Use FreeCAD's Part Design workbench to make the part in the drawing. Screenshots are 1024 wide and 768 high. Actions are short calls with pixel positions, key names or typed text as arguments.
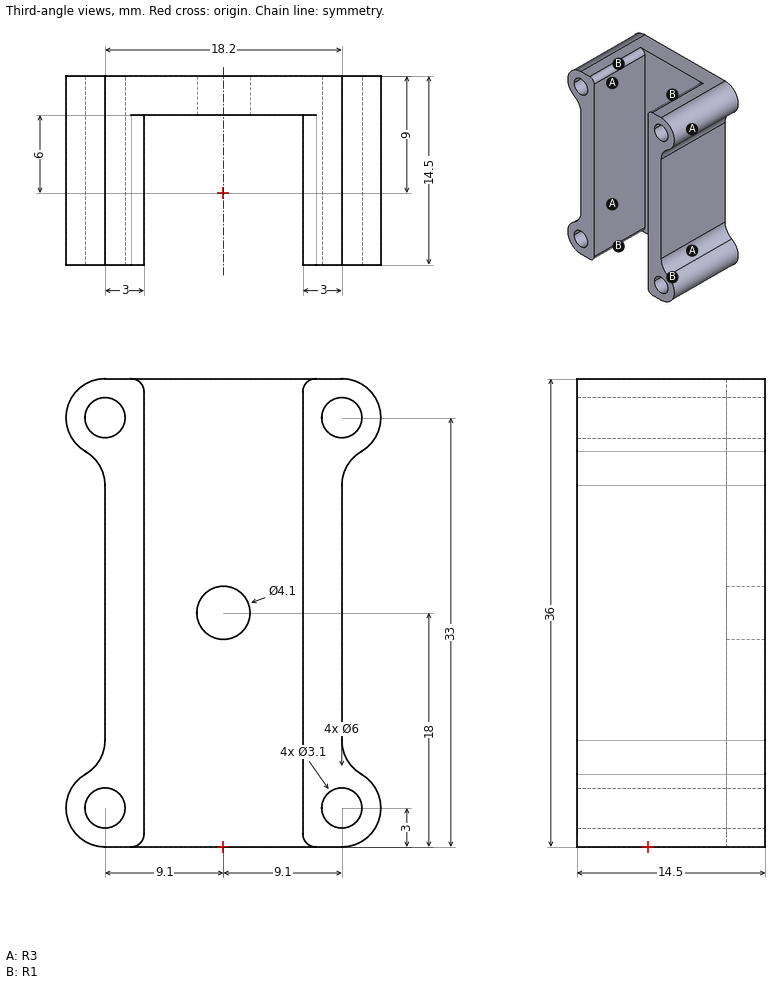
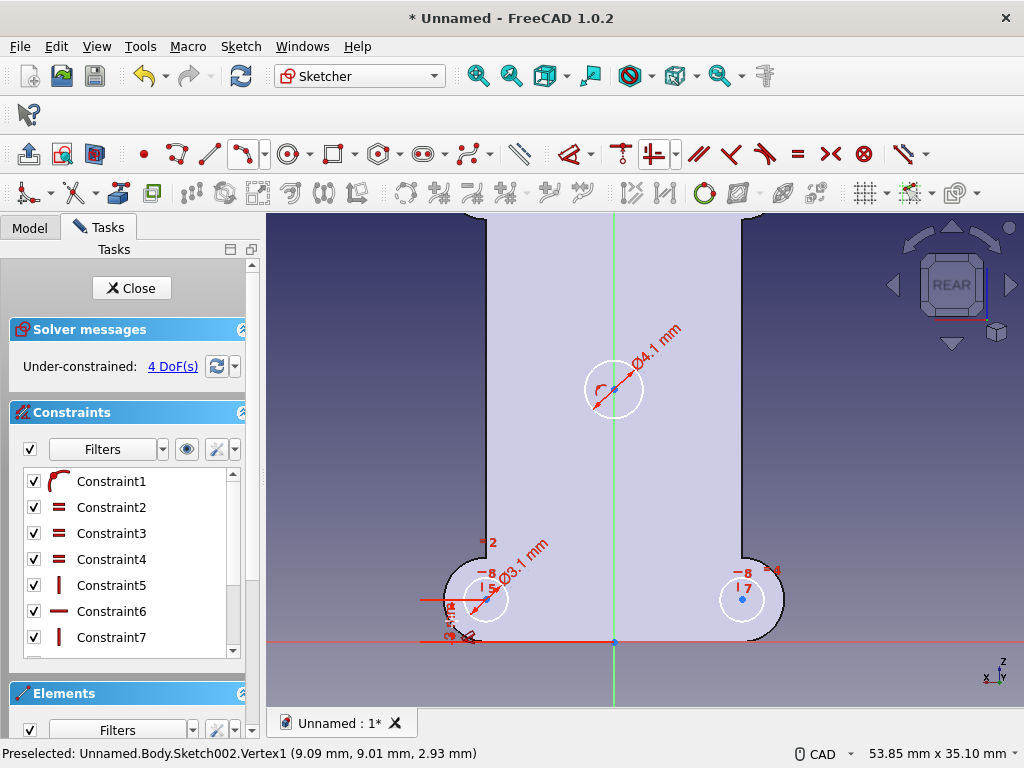
scroll(500, 584, down, 2)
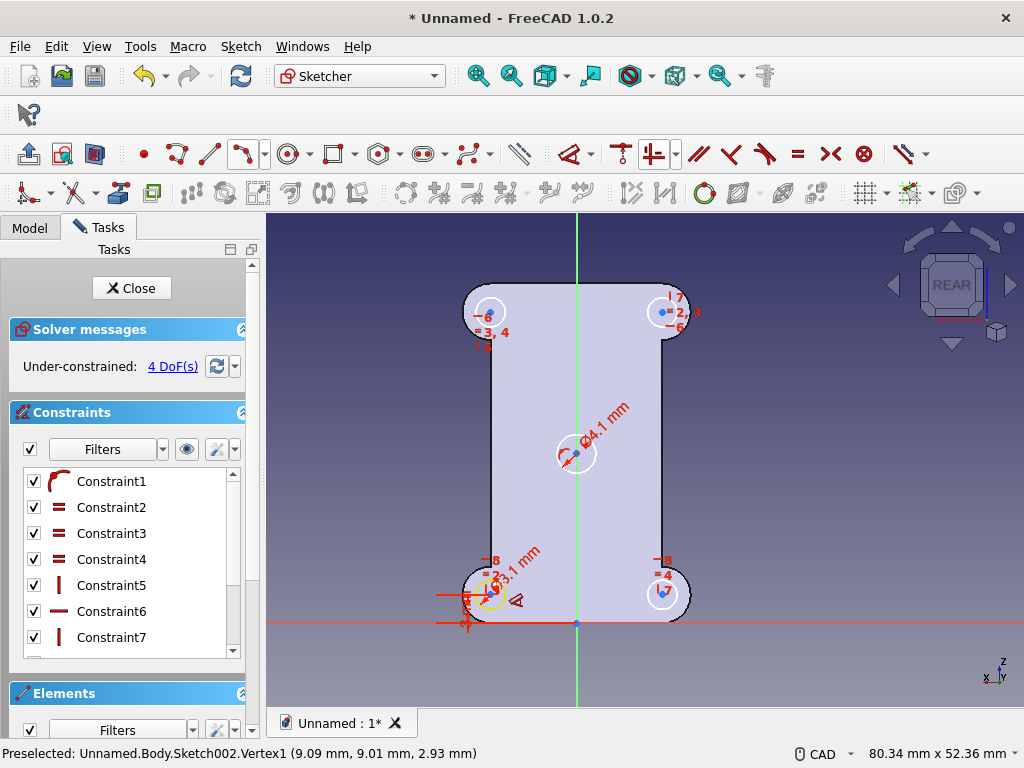
click(662, 312)
click(696, 468)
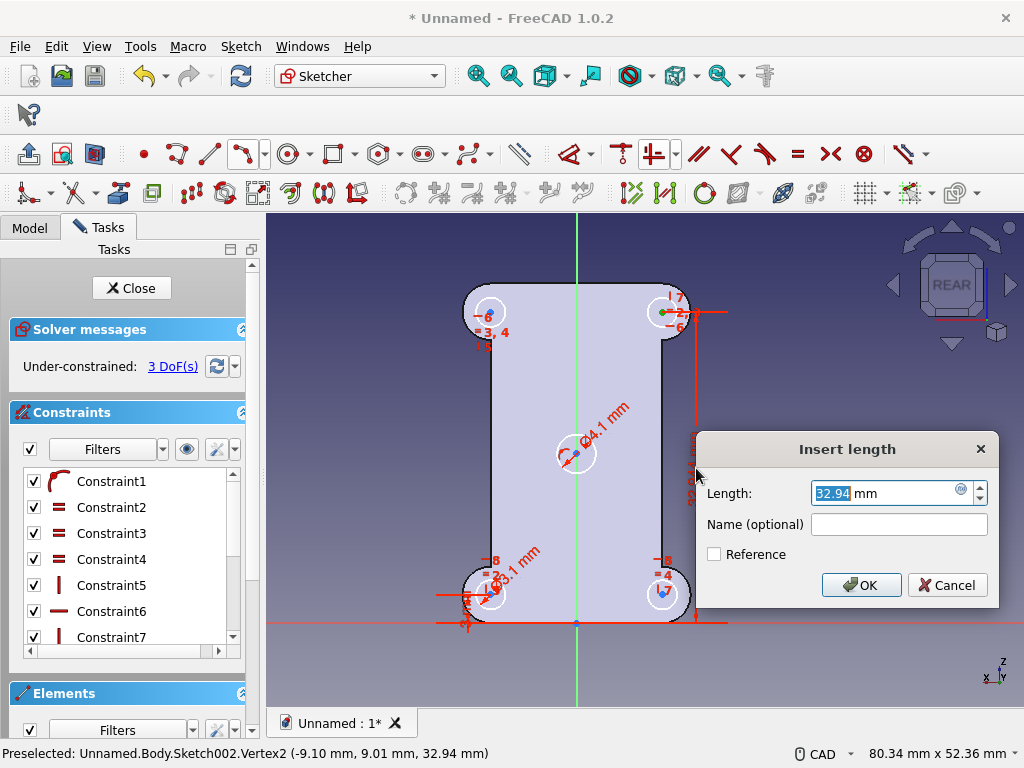
text(33)
key(Return)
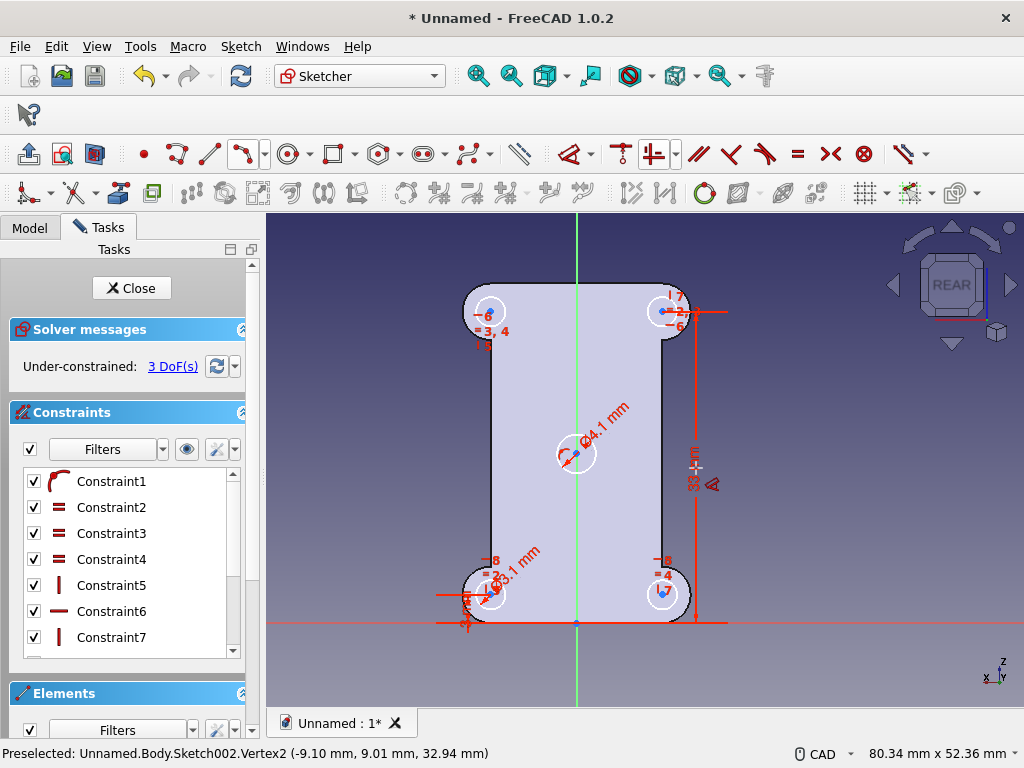
click(577, 454)
click(611, 539)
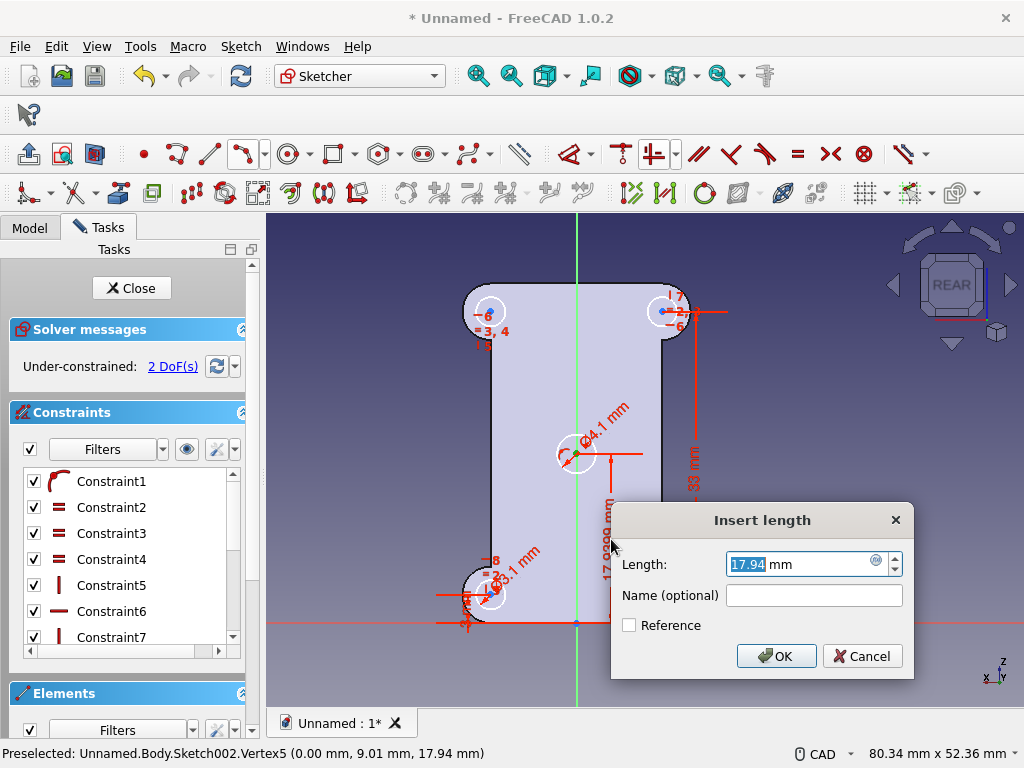
text(18)
key(Return)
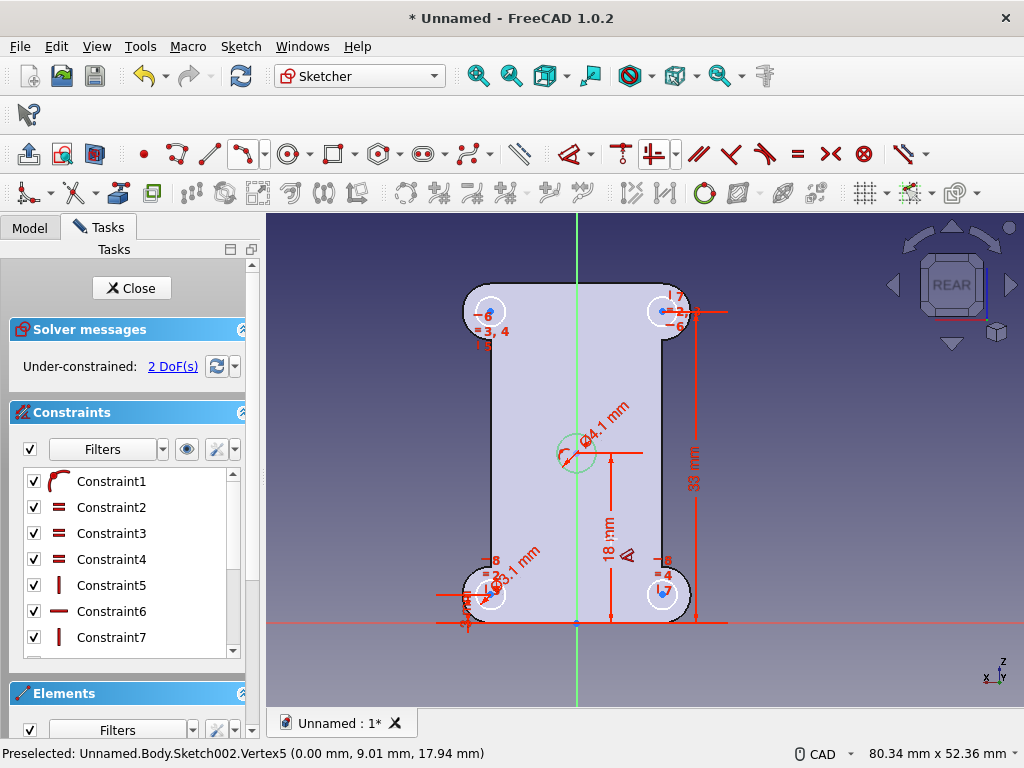
click(491, 595)
click(534, 657)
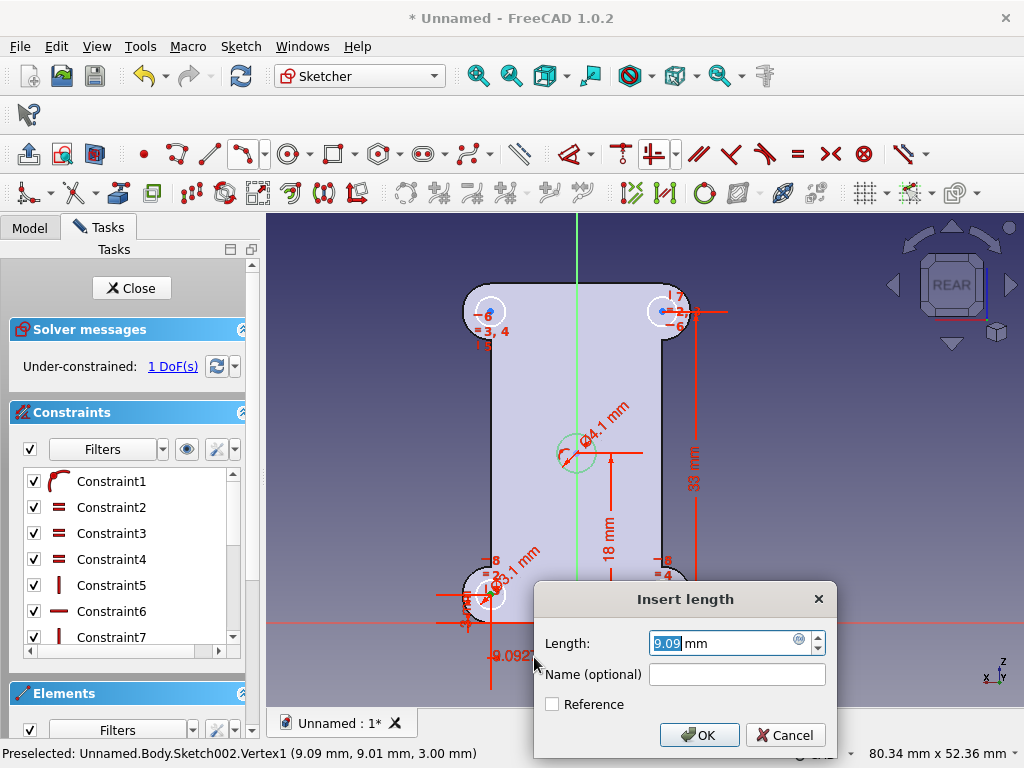
text(9.1)
key(Return)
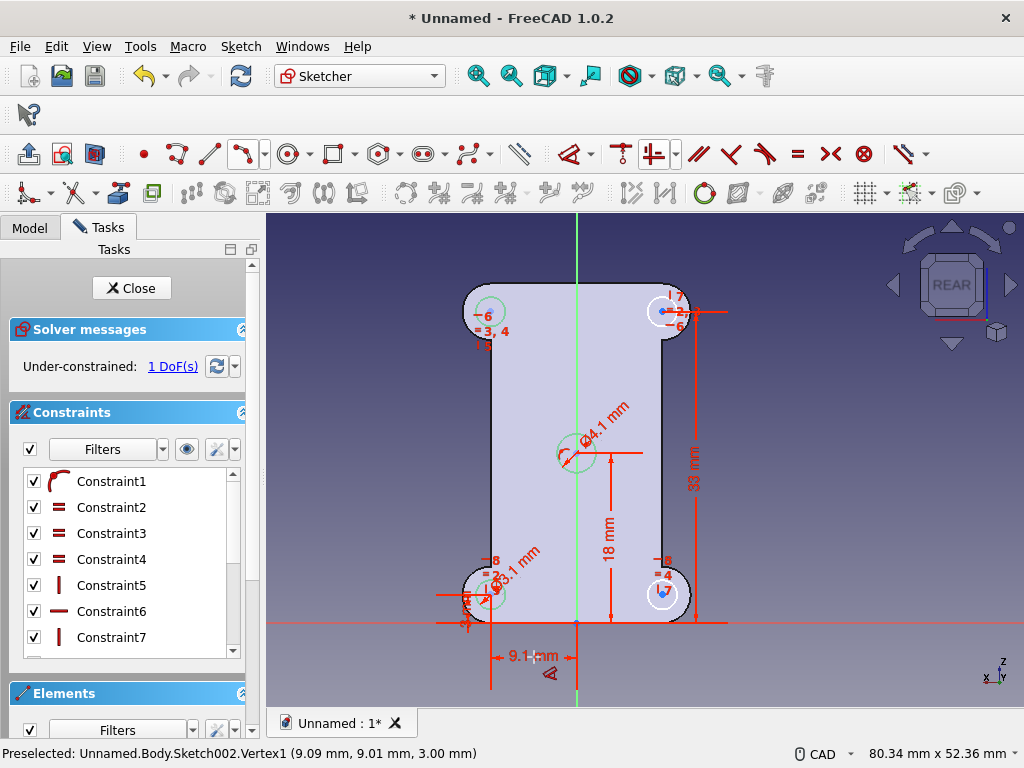
click(662, 312)
click(619, 657)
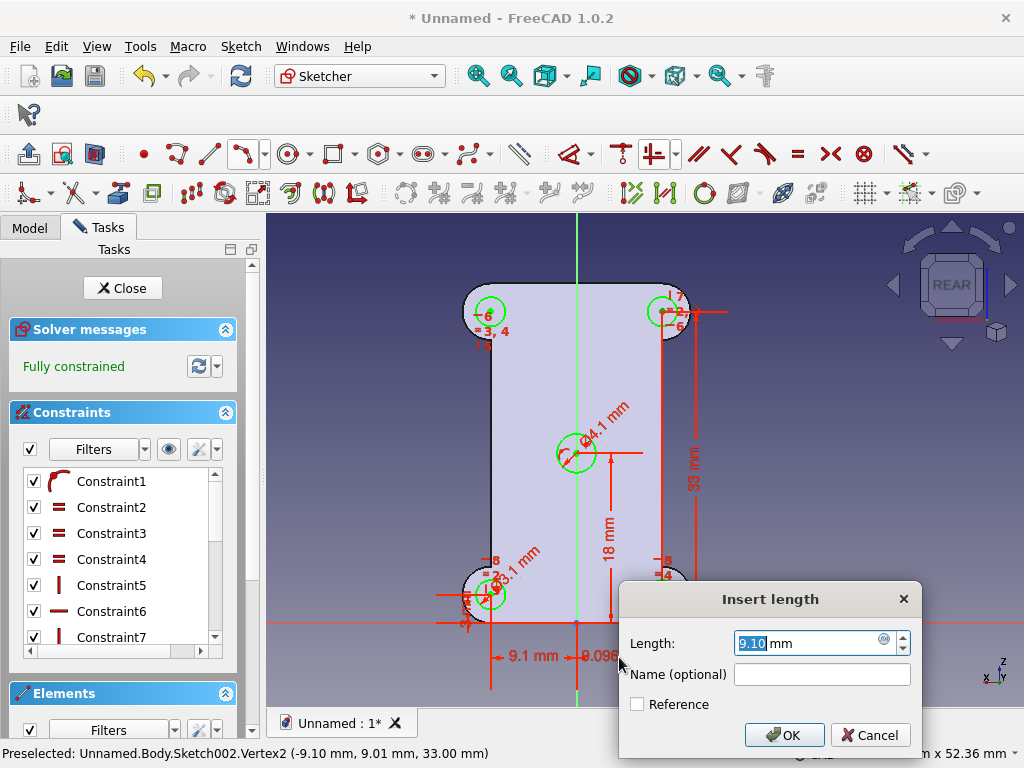
text(9.1)
key(Return)
key(Escape)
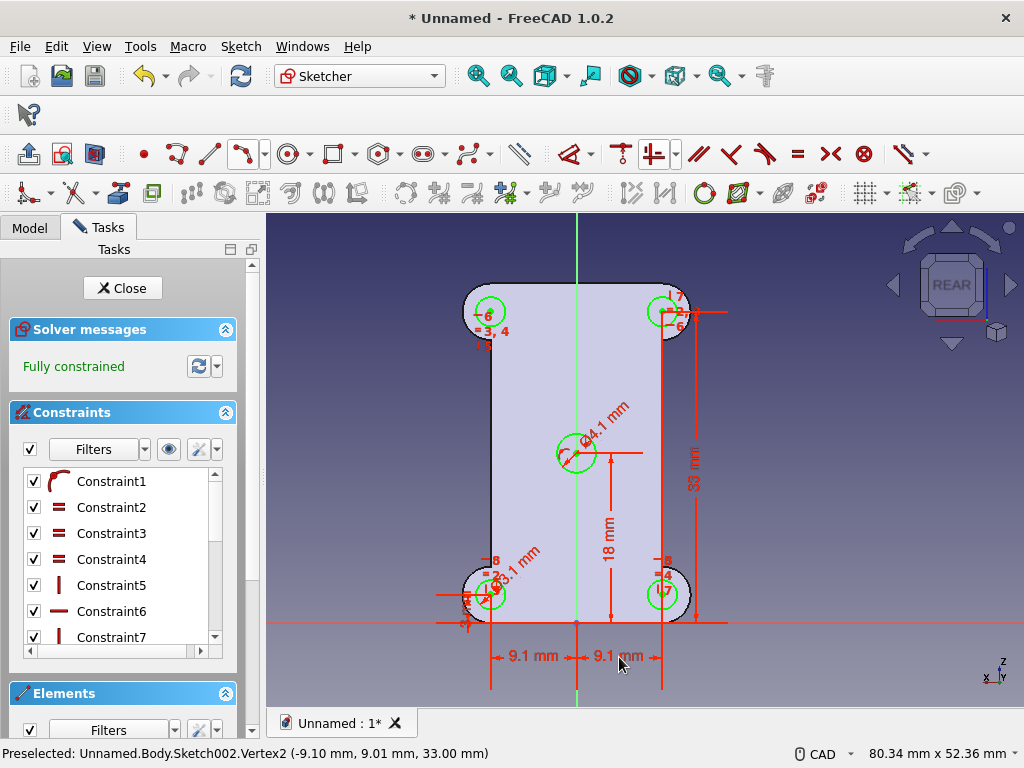
click(123, 288)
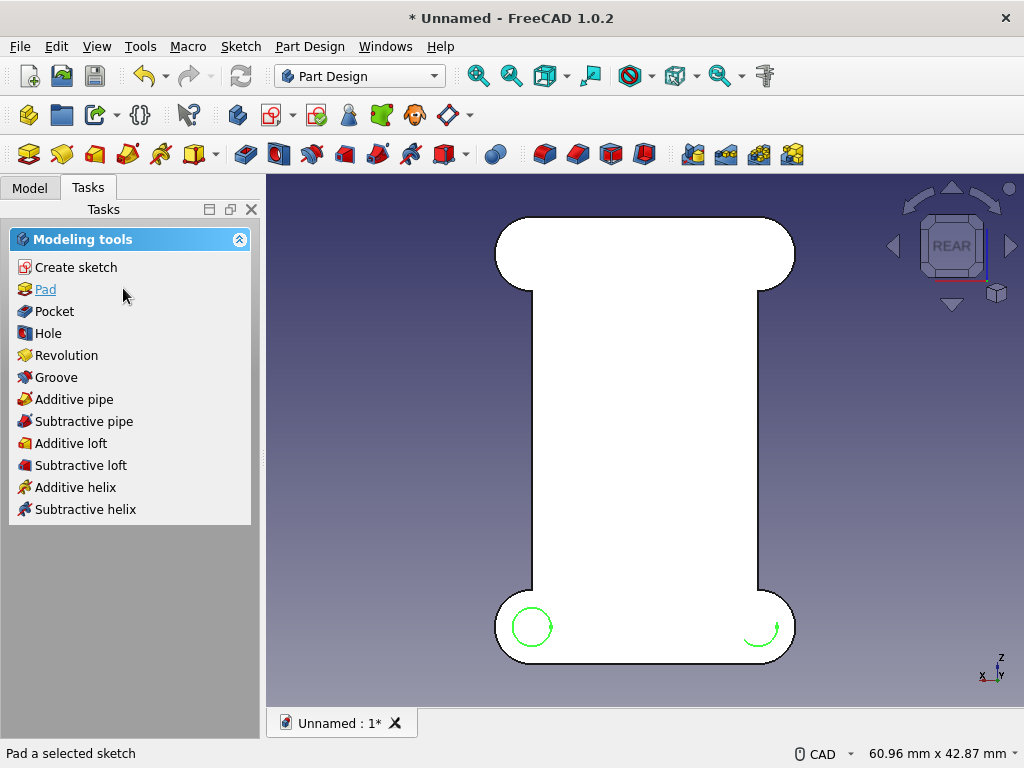
click(246, 154)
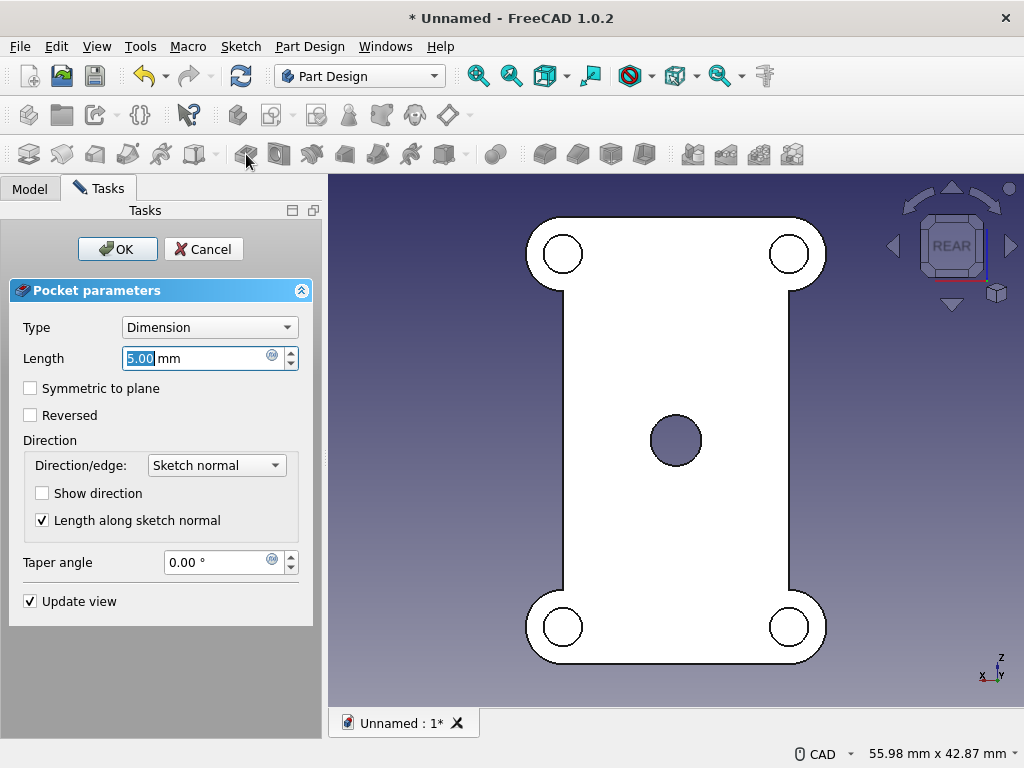
click(210, 328)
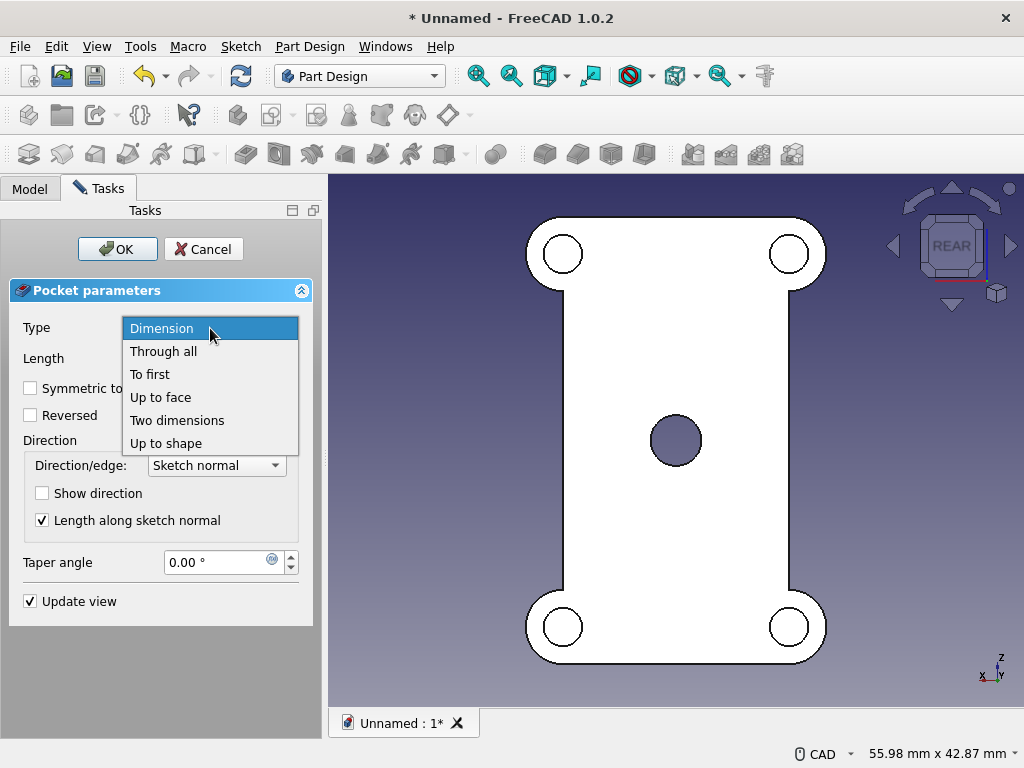
click(208, 352)